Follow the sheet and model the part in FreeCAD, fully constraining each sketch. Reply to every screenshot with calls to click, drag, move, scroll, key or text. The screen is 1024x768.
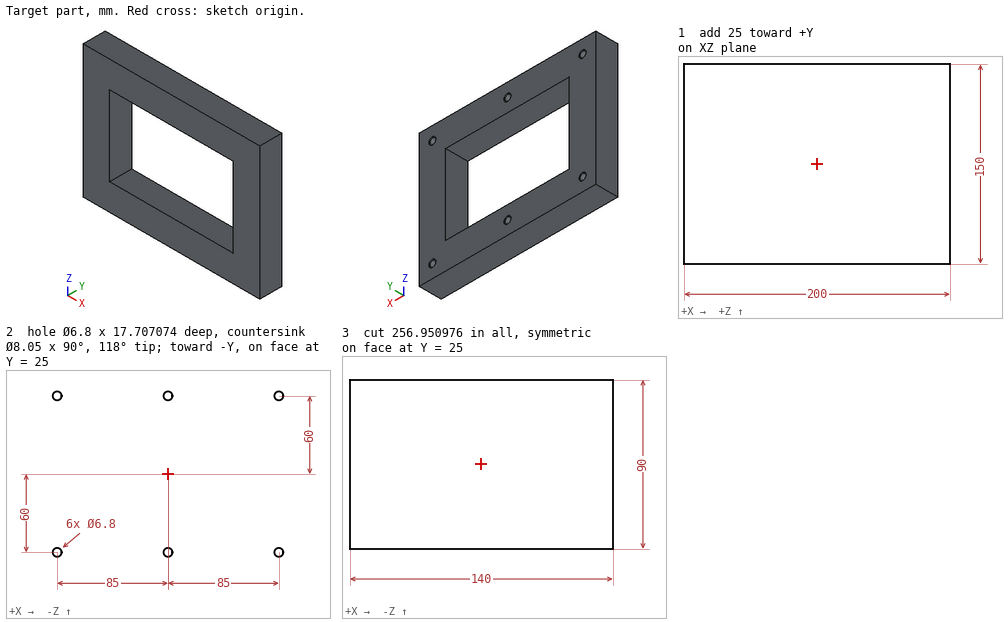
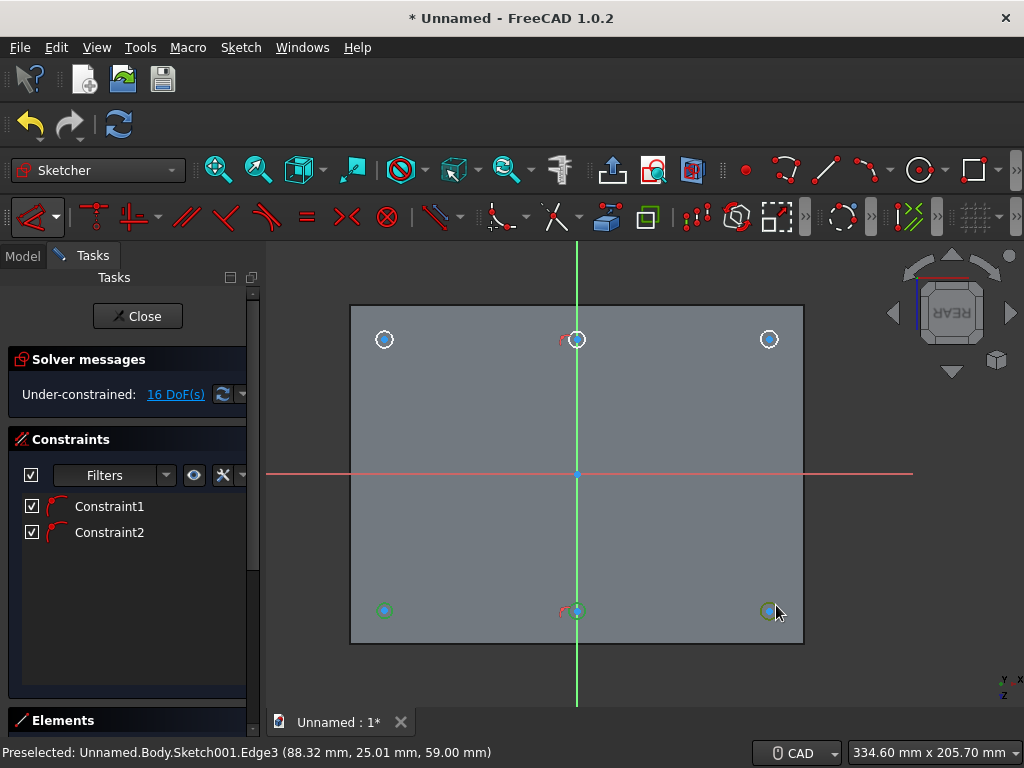
scroll(775, 333, up, 3)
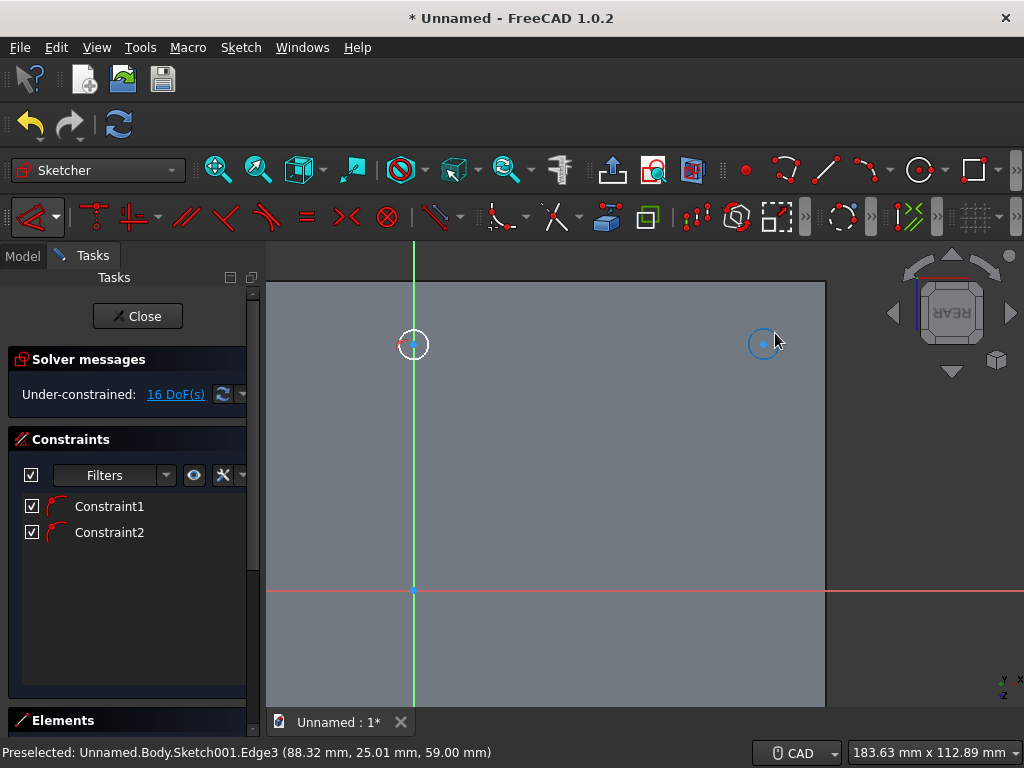
click(775, 333)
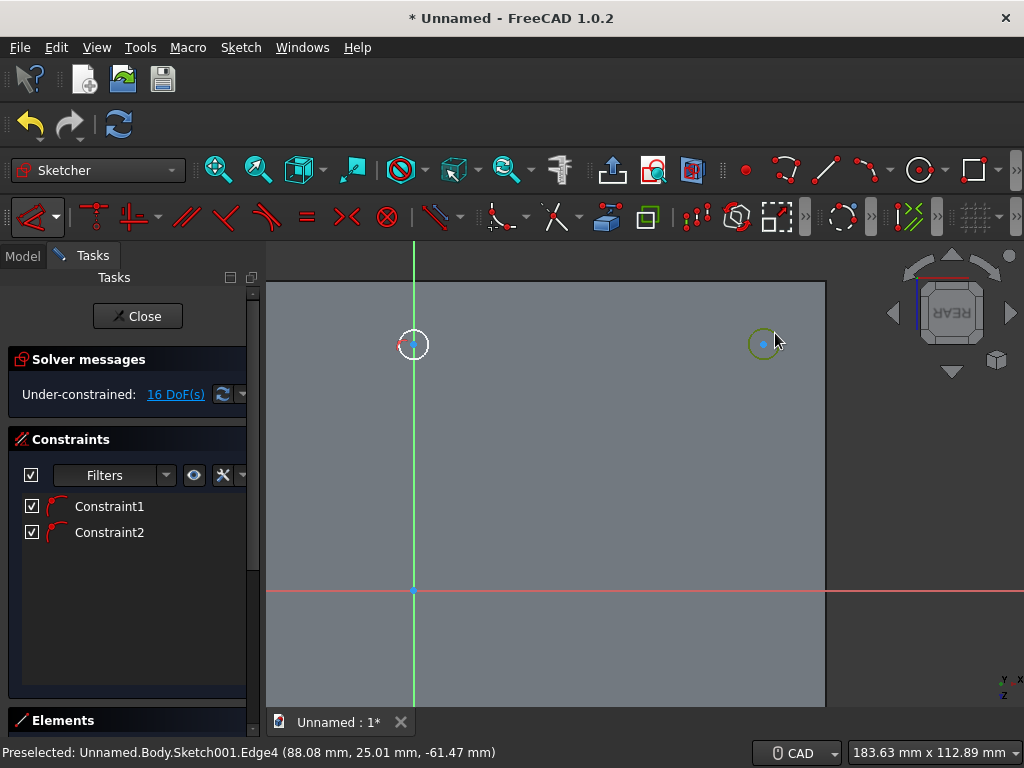
scroll(424, 334, up, 2)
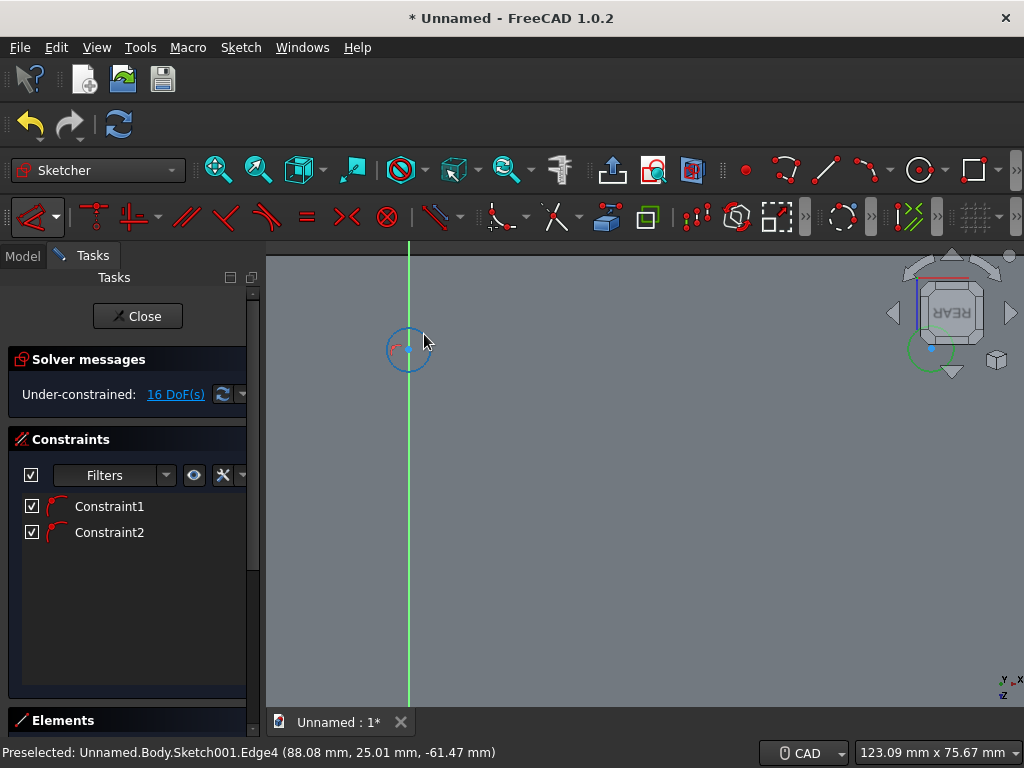
click(424, 335)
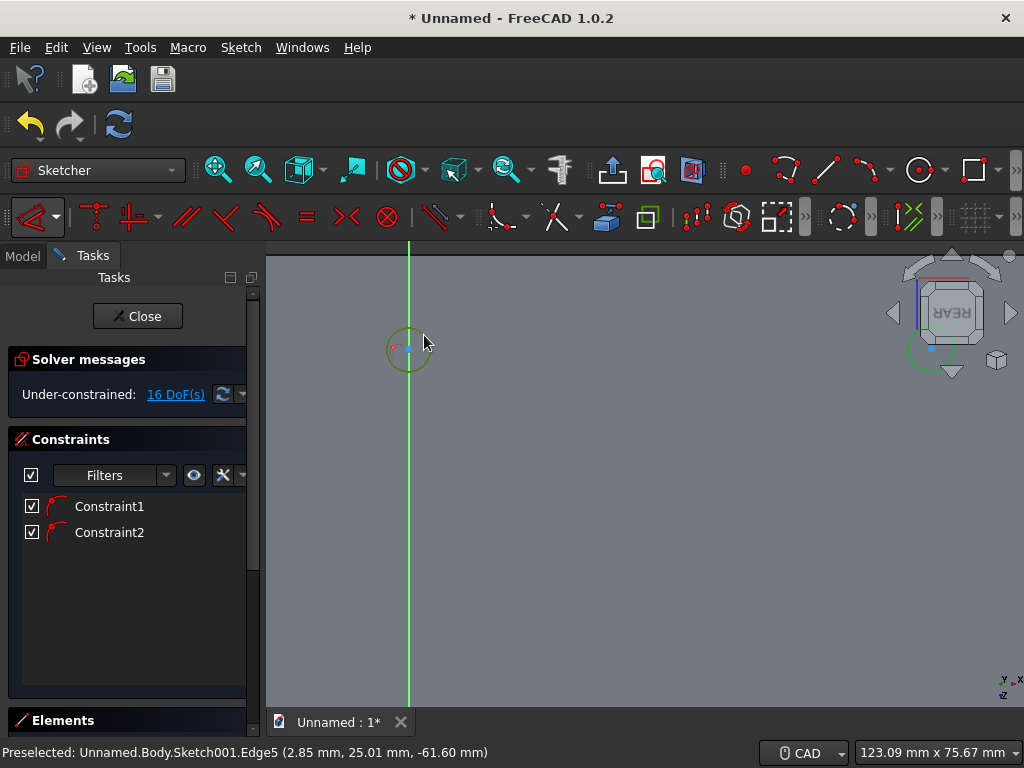
scroll(674, 333, down, 5)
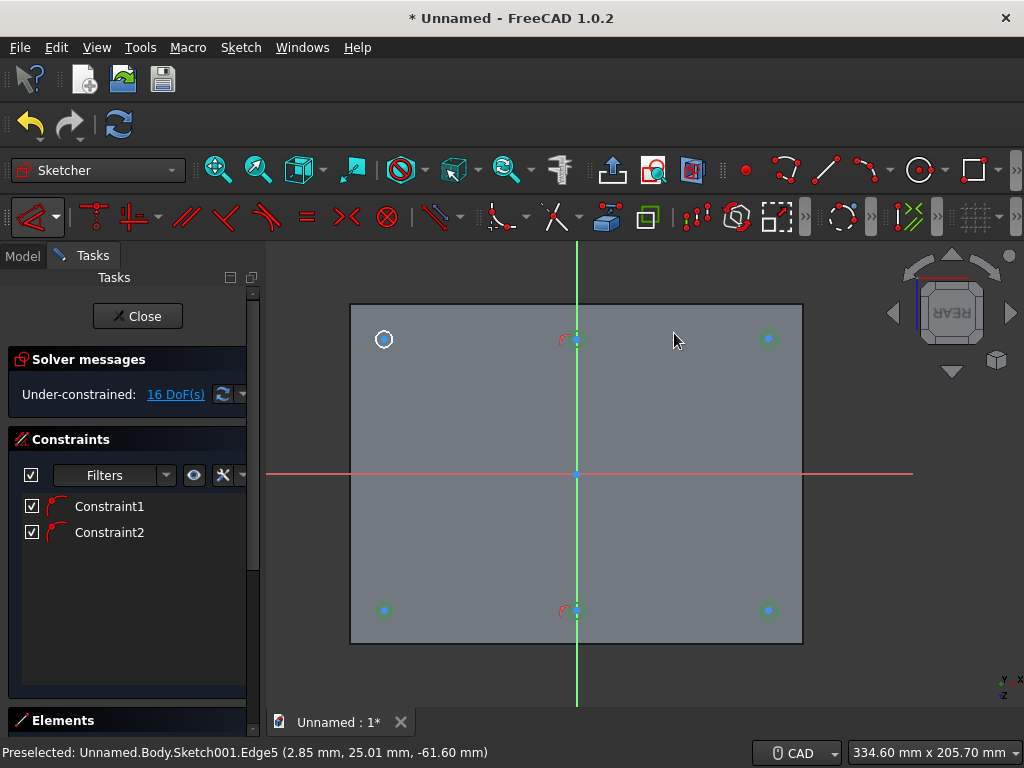
scroll(390, 334, up, 3)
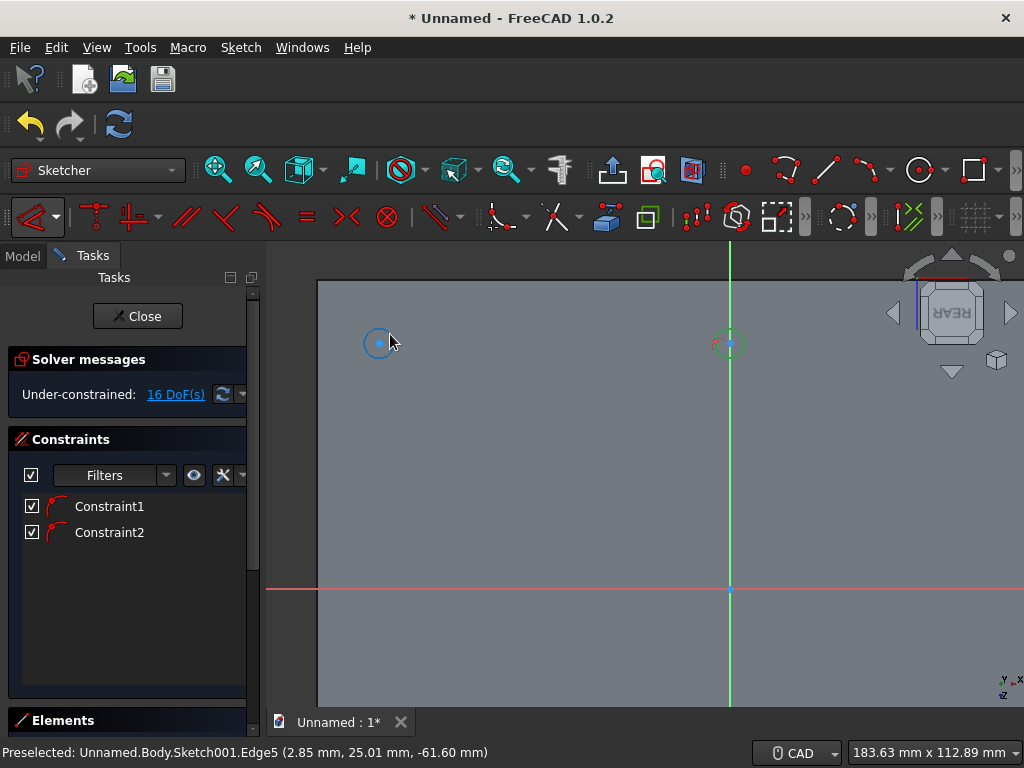
click(390, 333)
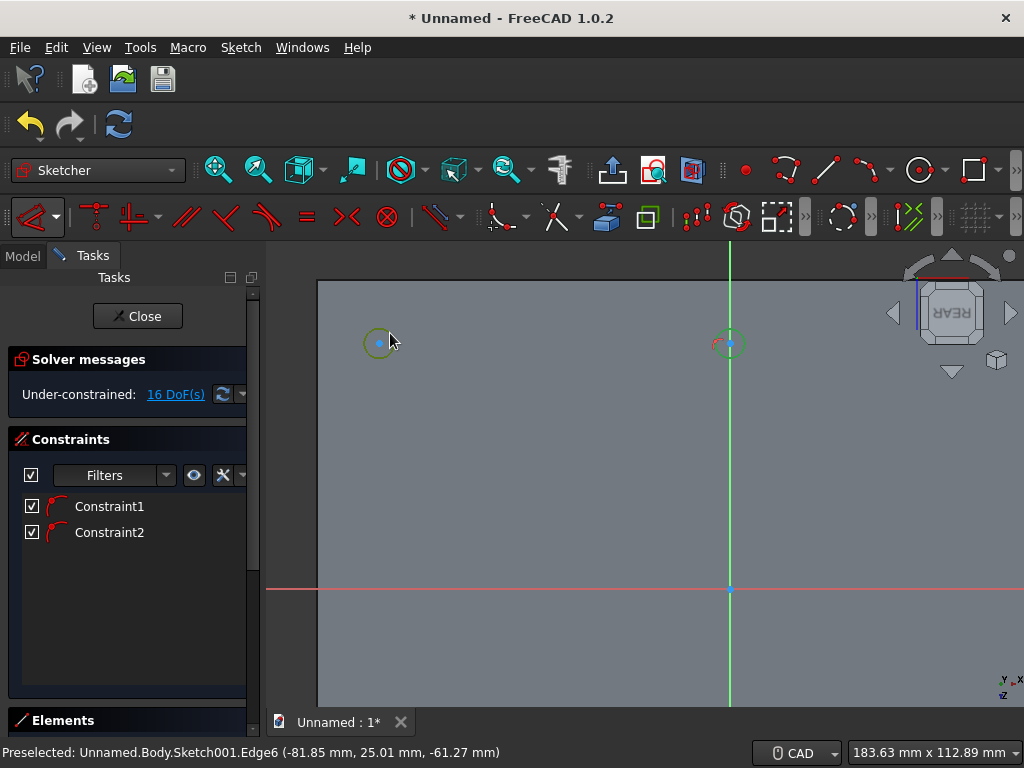
click(308, 218)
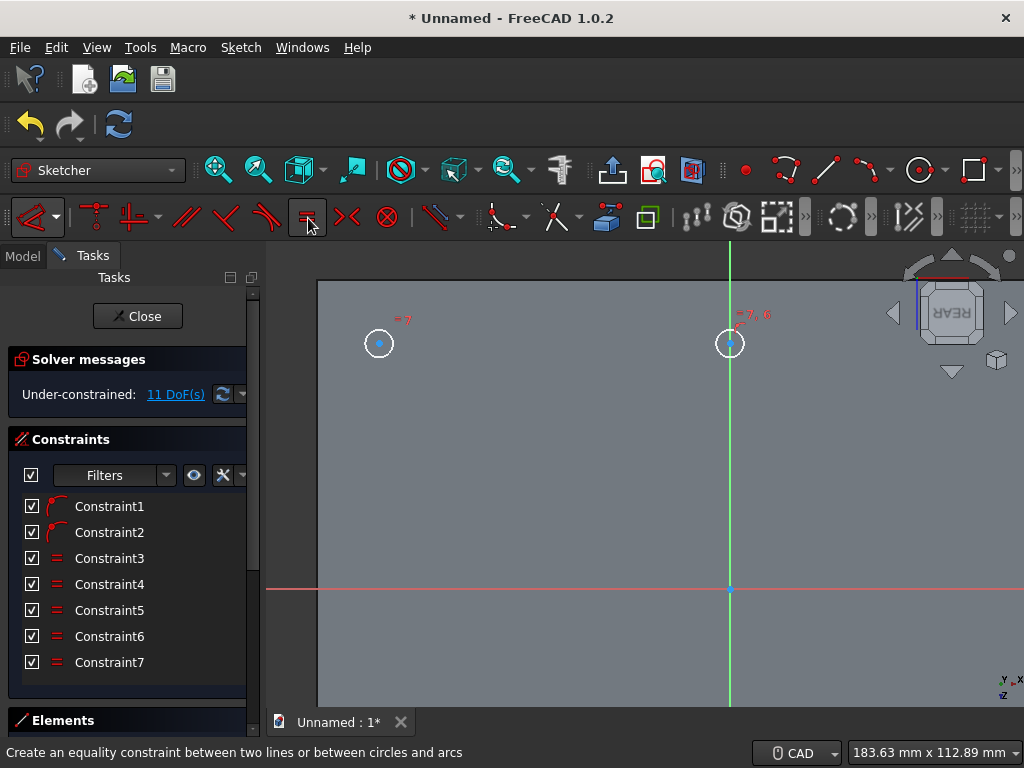
scroll(390, 334, down, 3)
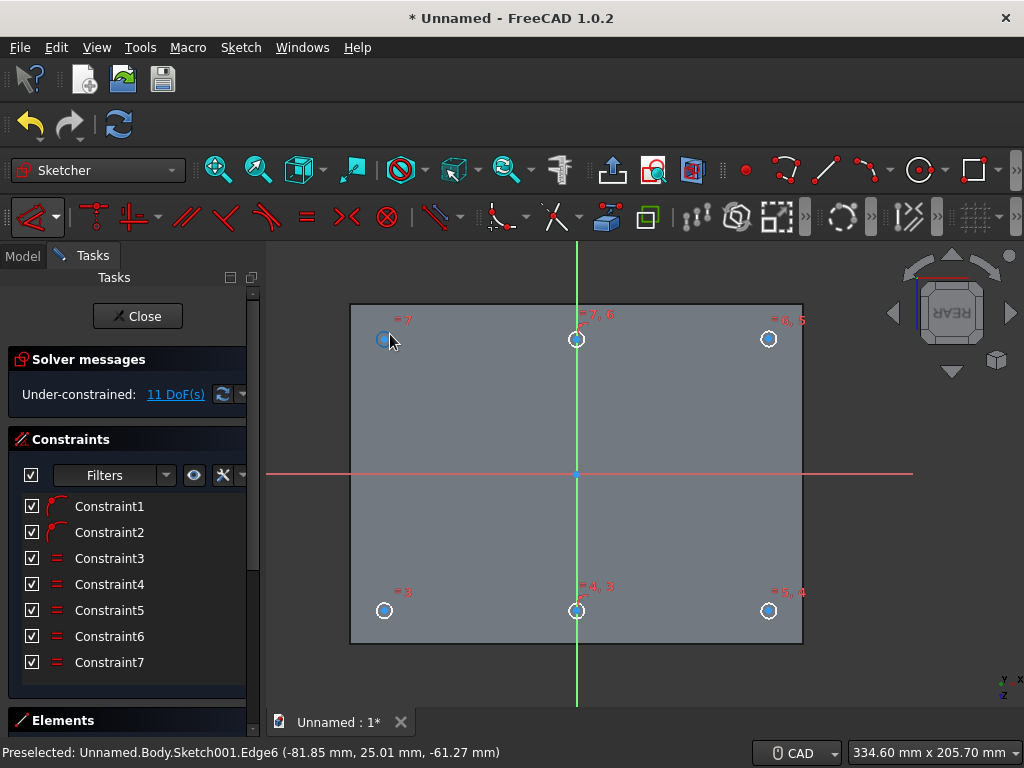
click(384, 611)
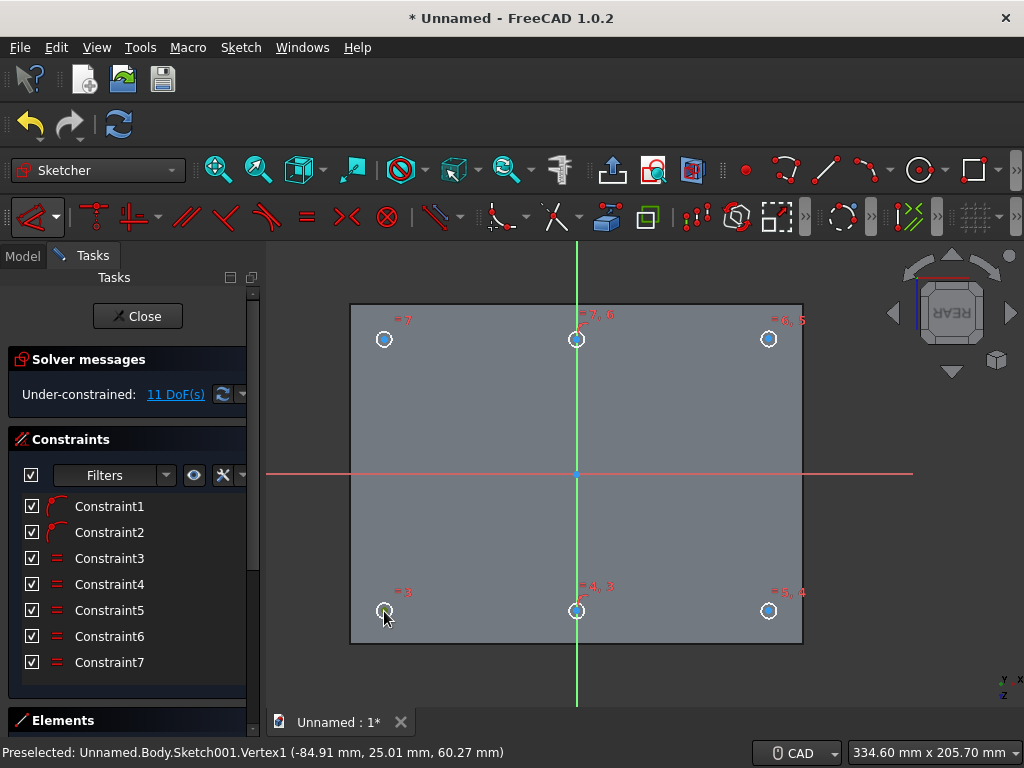
click(577, 611)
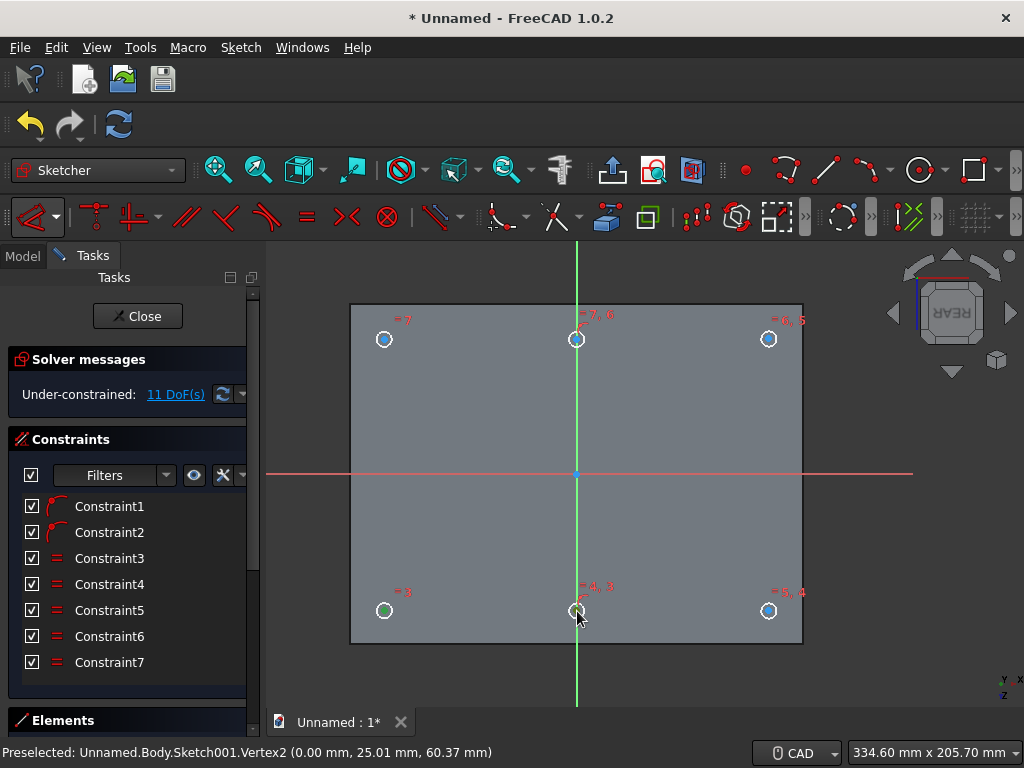
key(h)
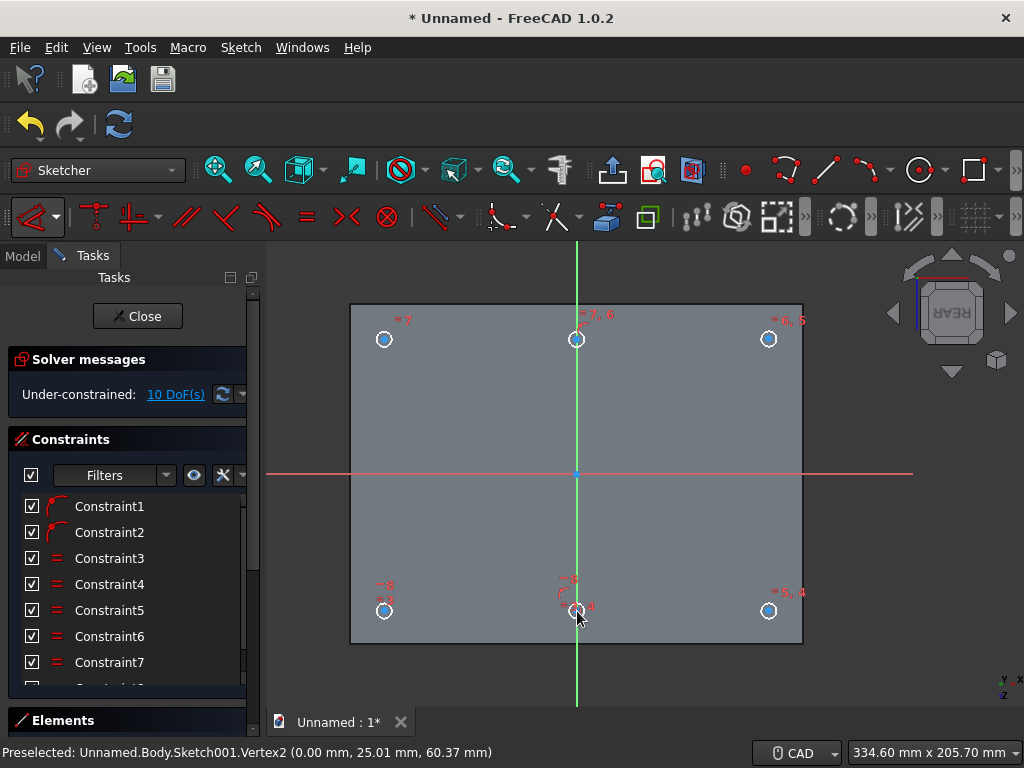
click(575, 613)